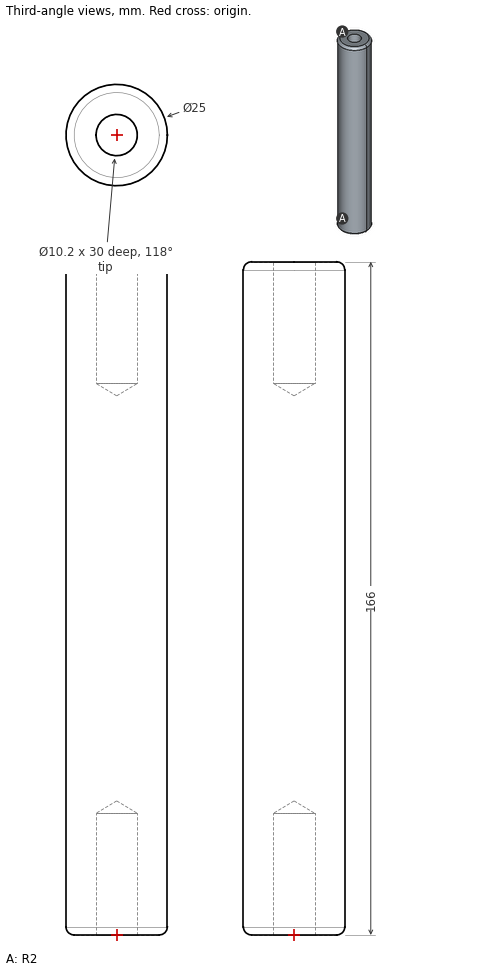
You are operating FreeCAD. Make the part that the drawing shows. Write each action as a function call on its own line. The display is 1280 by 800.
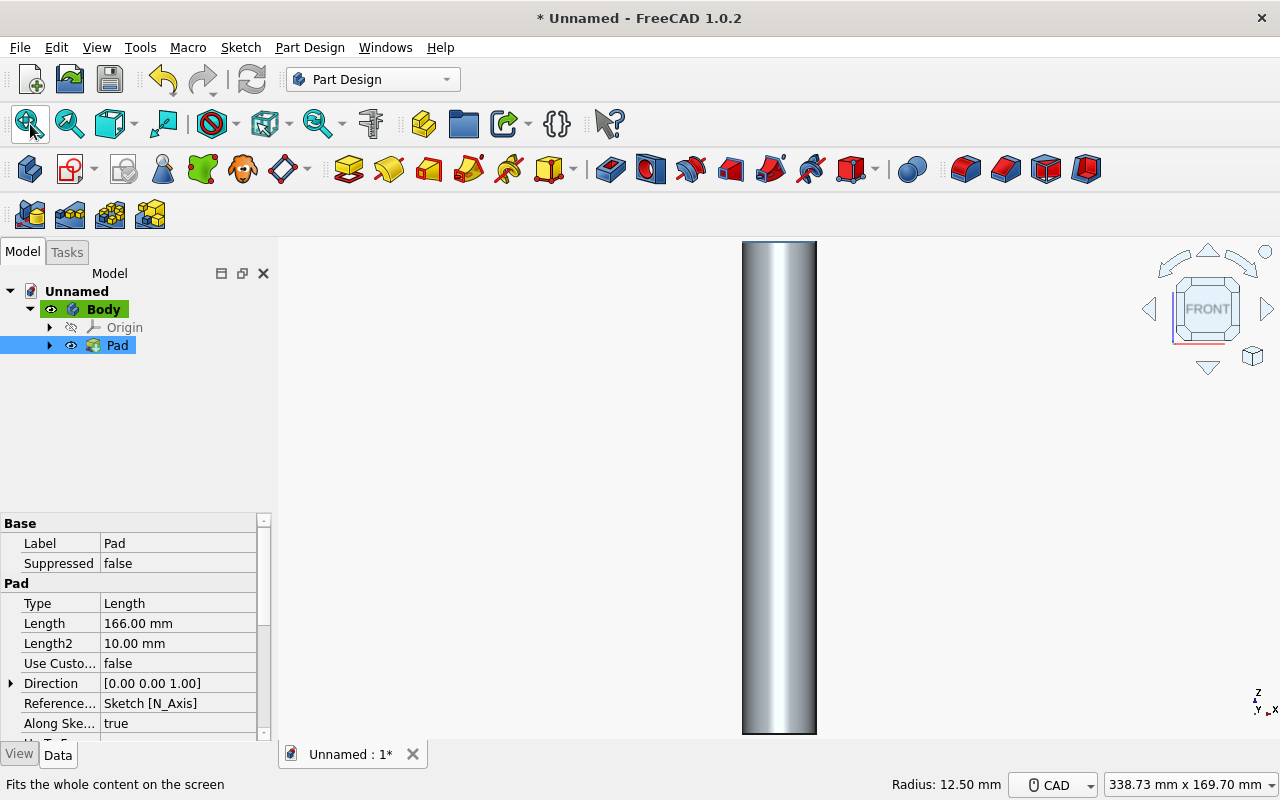
key(3)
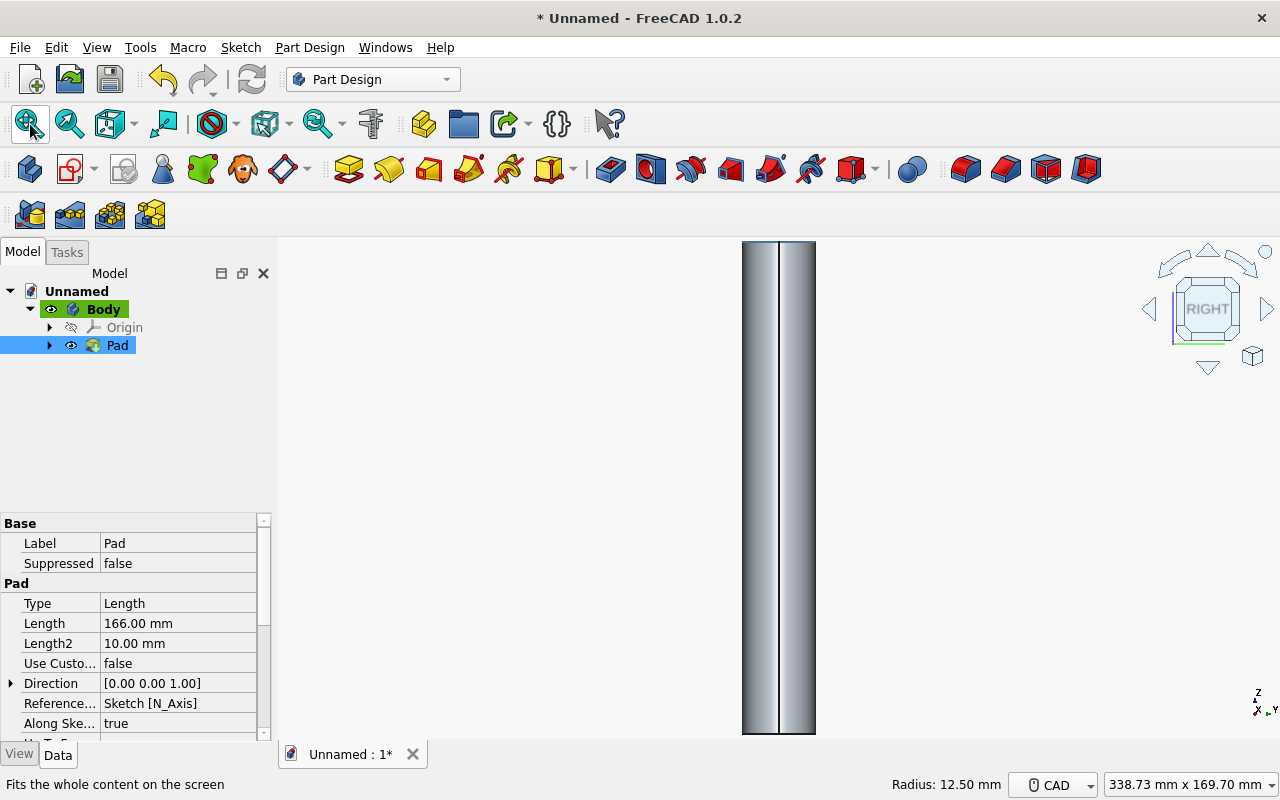
key(5)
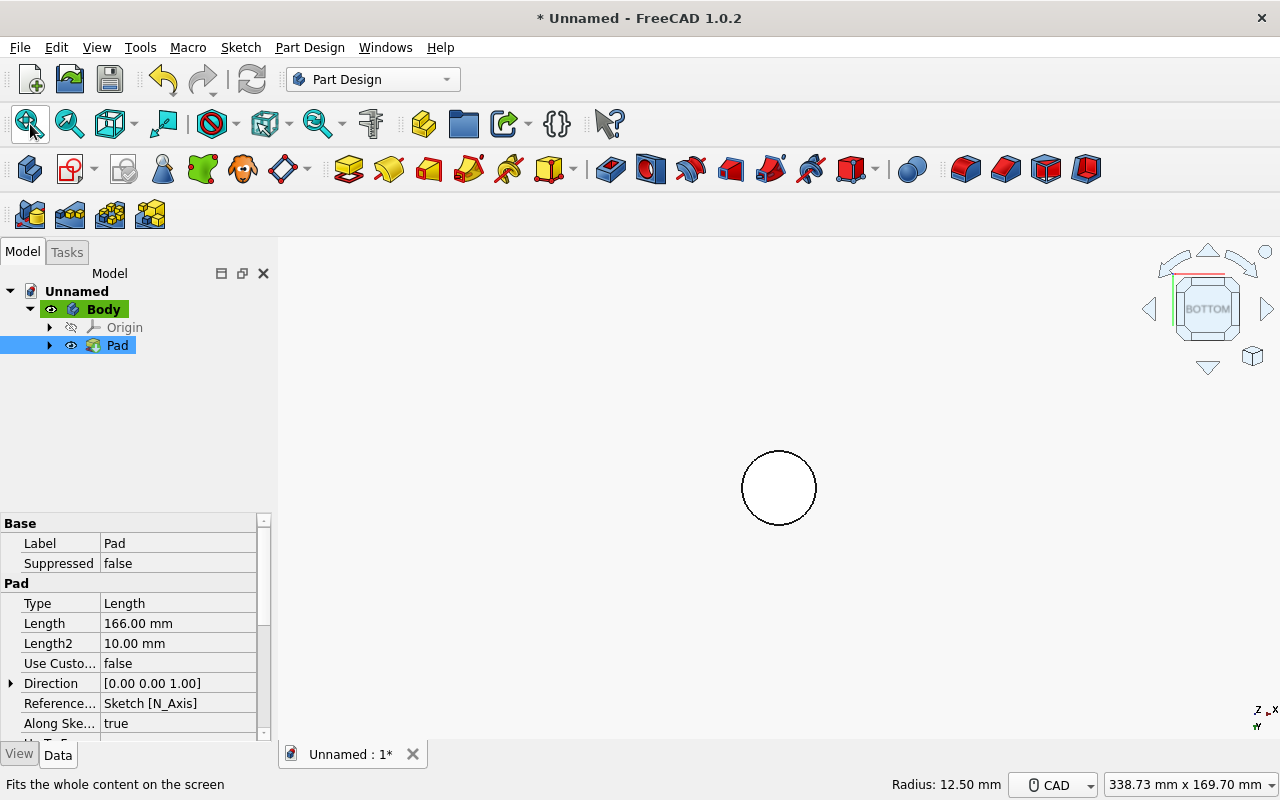
click(30, 124)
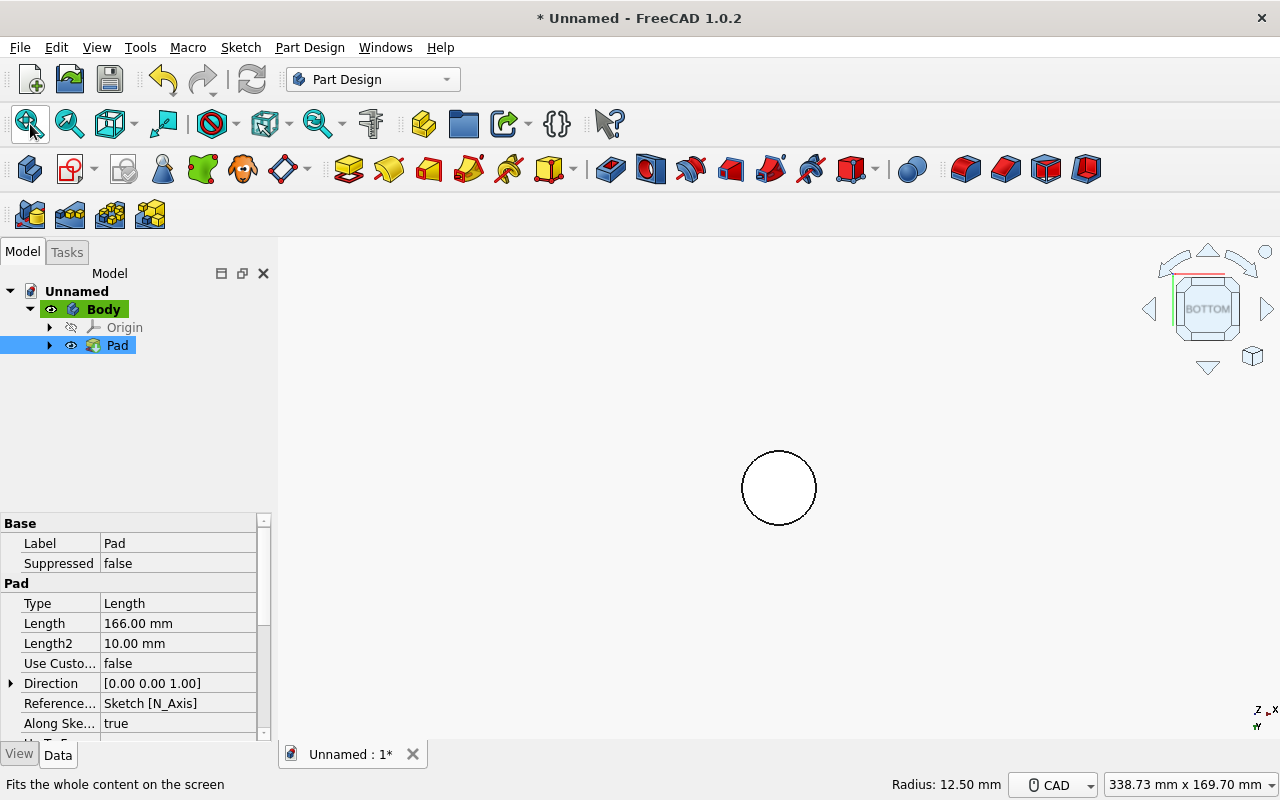
click(742, 487, ctrl)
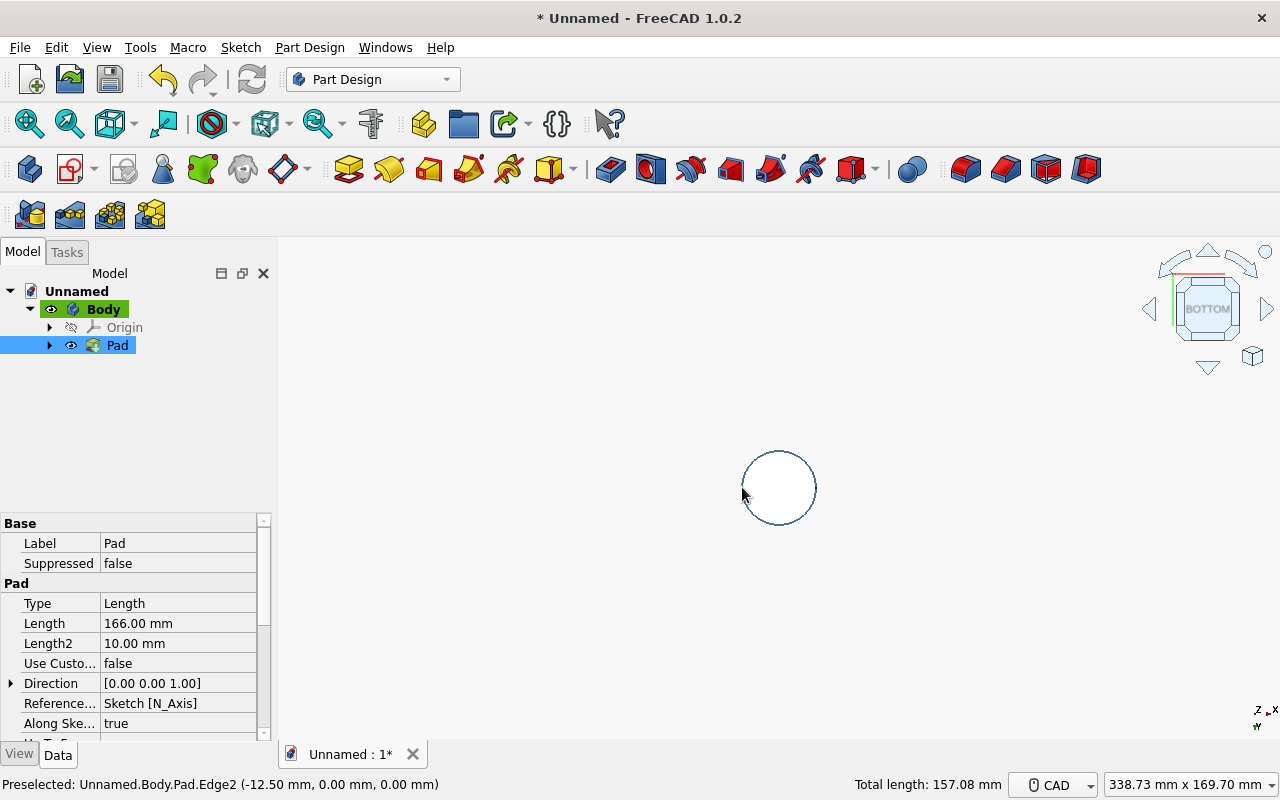
click(966, 170)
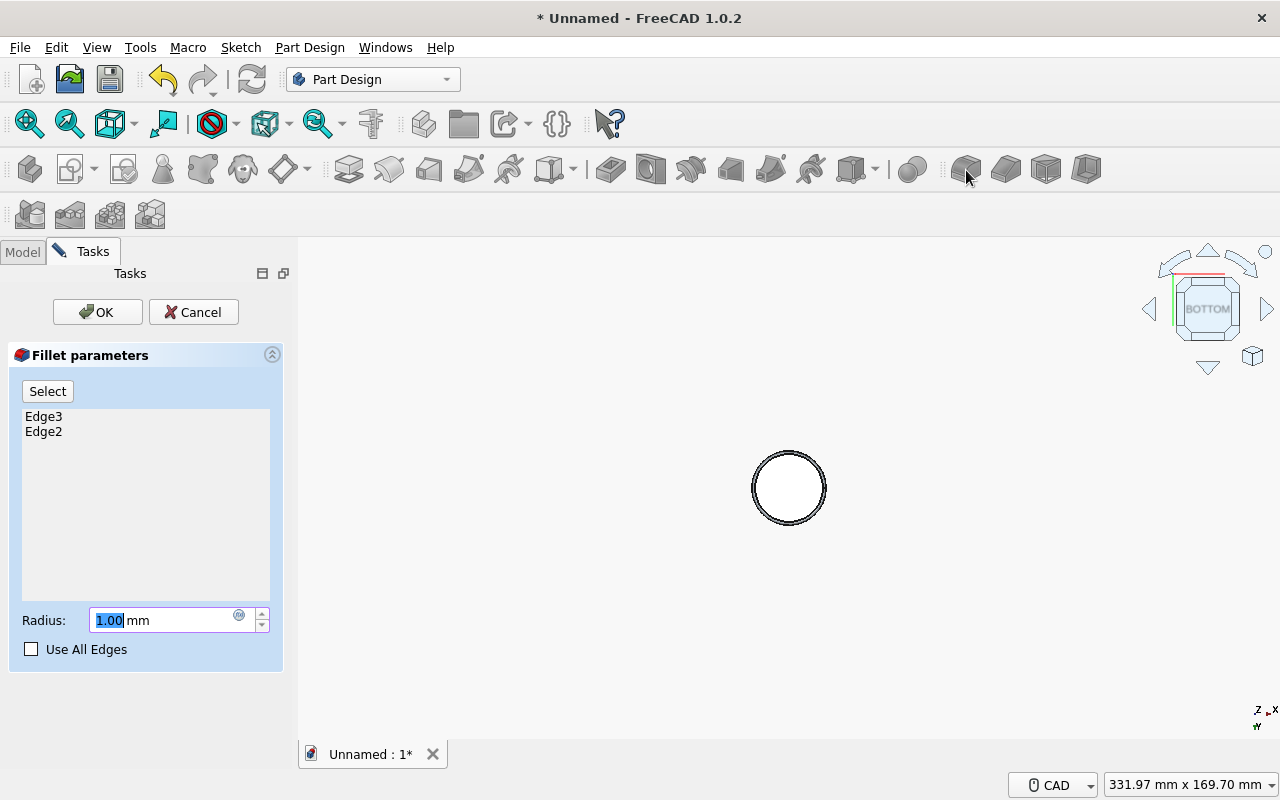
text(2)
key(Tab)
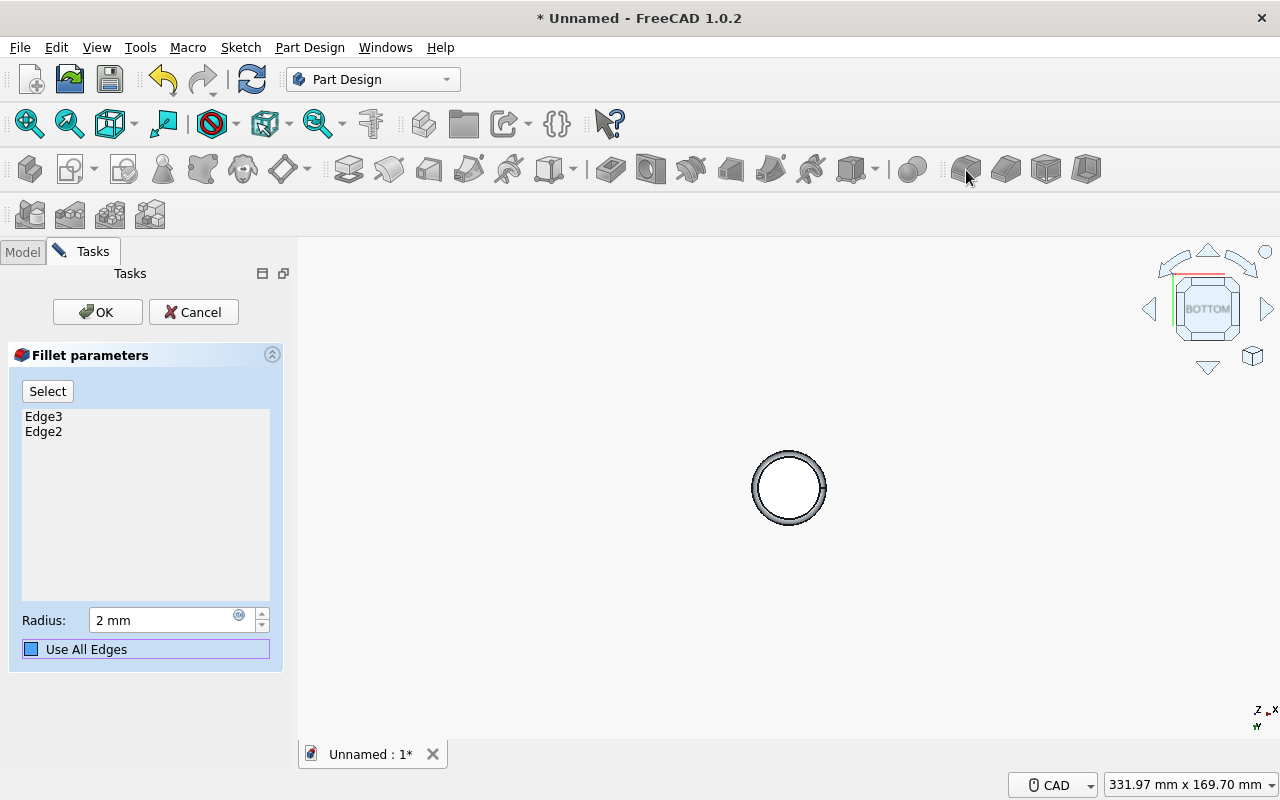
click(98, 312)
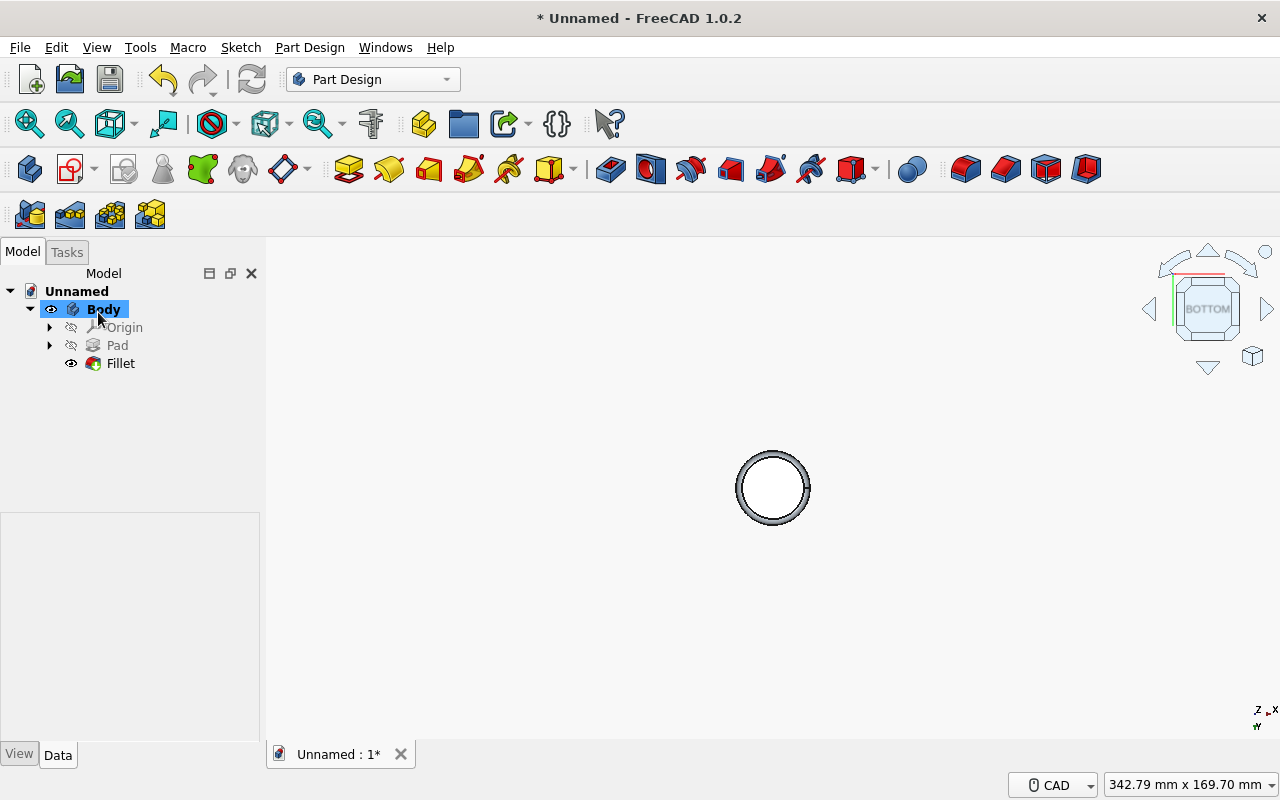
click(30, 124)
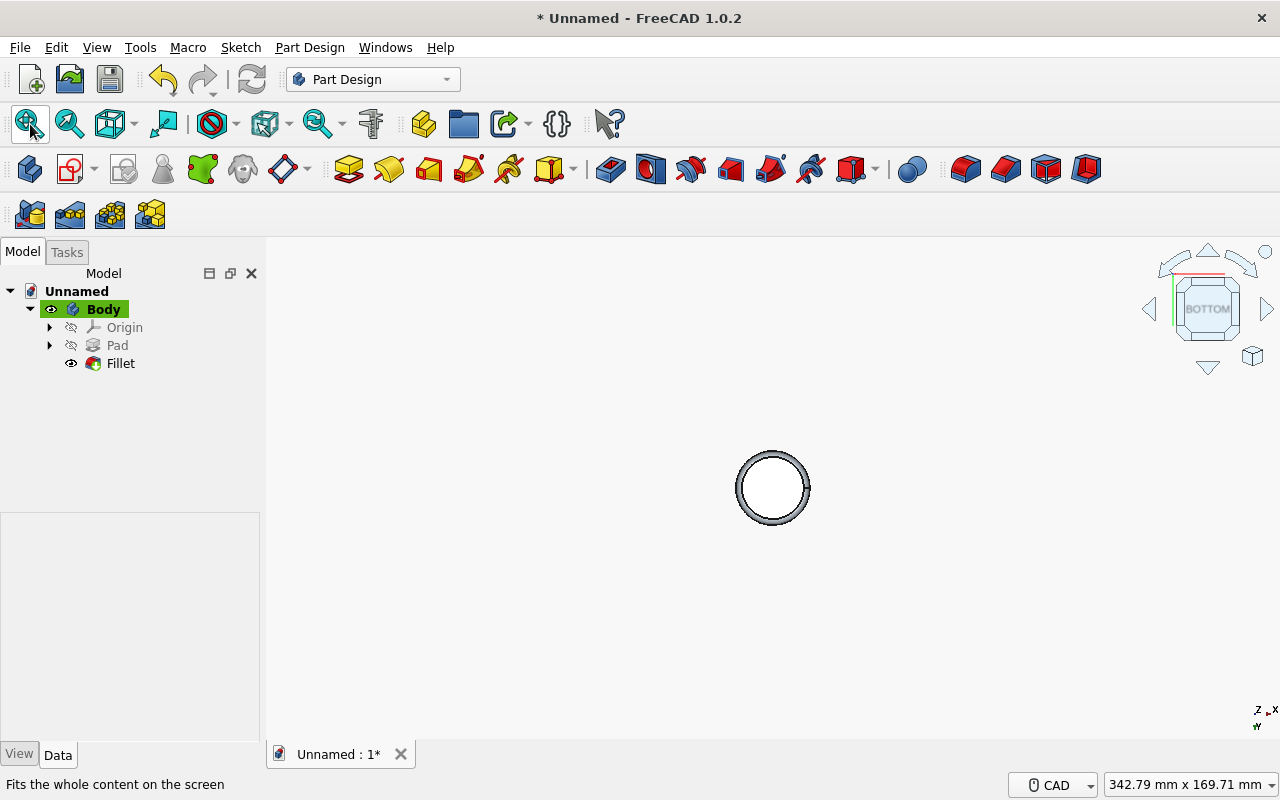
key(0)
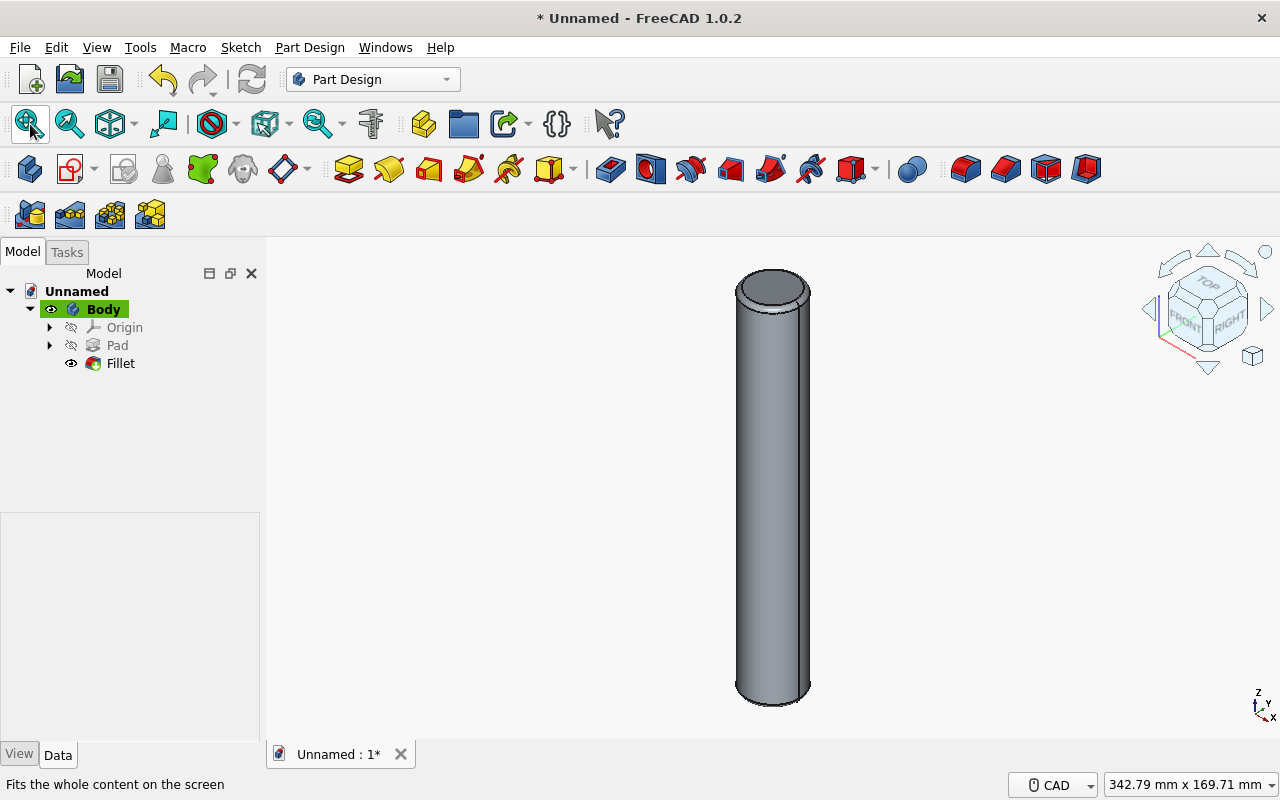
click(773, 286)